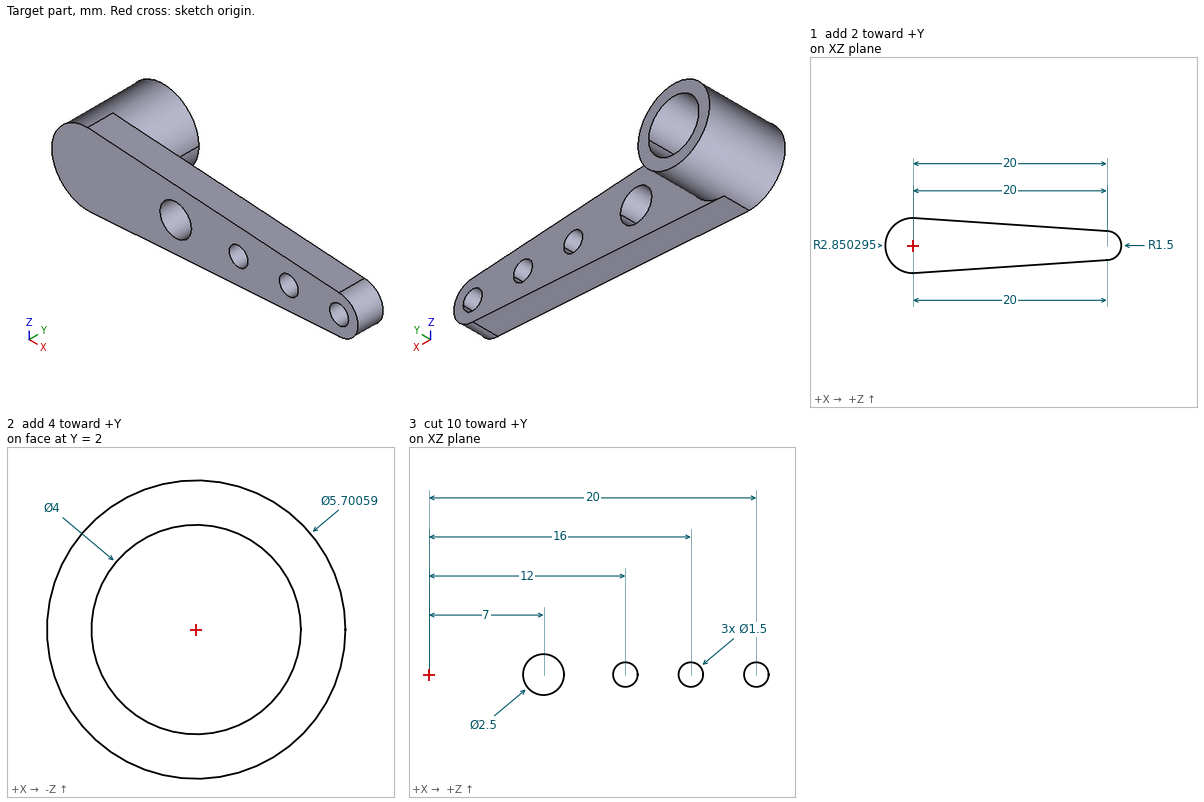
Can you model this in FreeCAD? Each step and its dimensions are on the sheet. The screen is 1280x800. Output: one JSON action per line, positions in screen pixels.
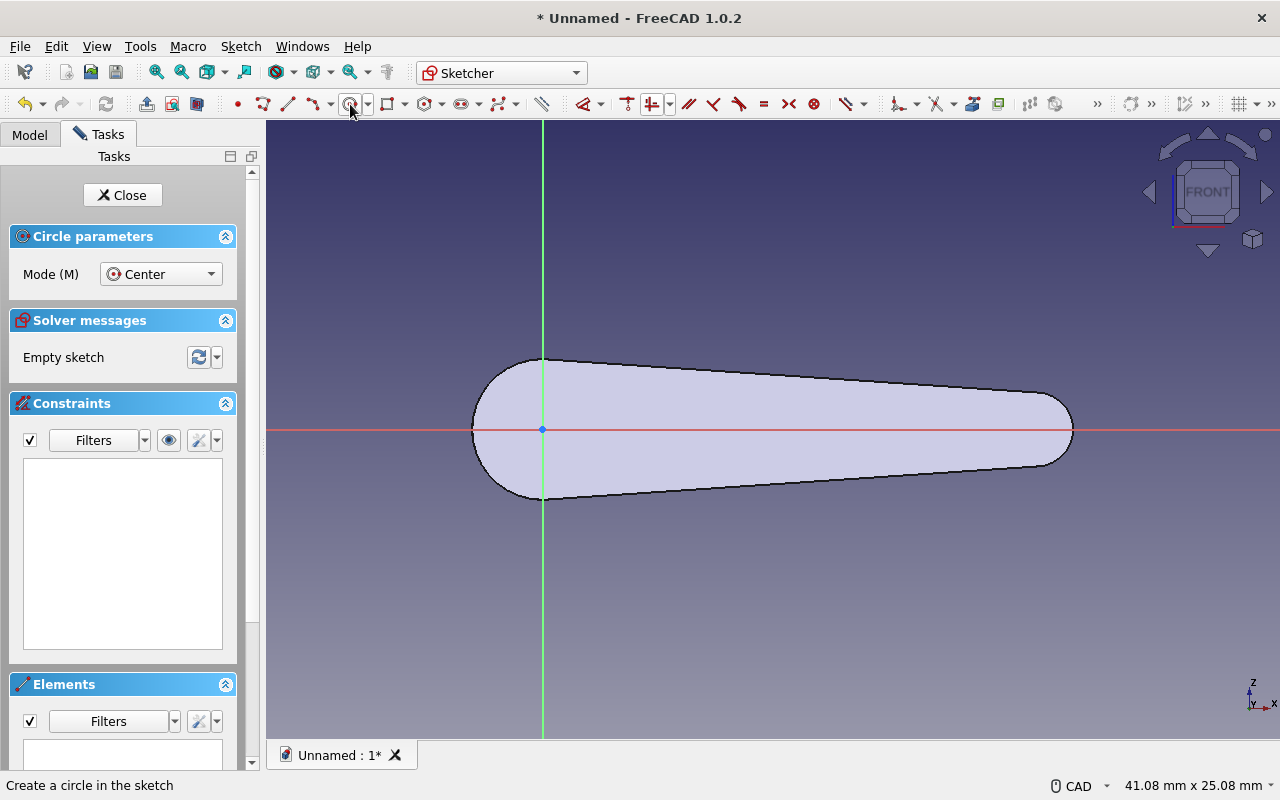
{"action": "scroll", "coordinate": [937, 430], "scroll_direction": "up", "scroll_amount": 2}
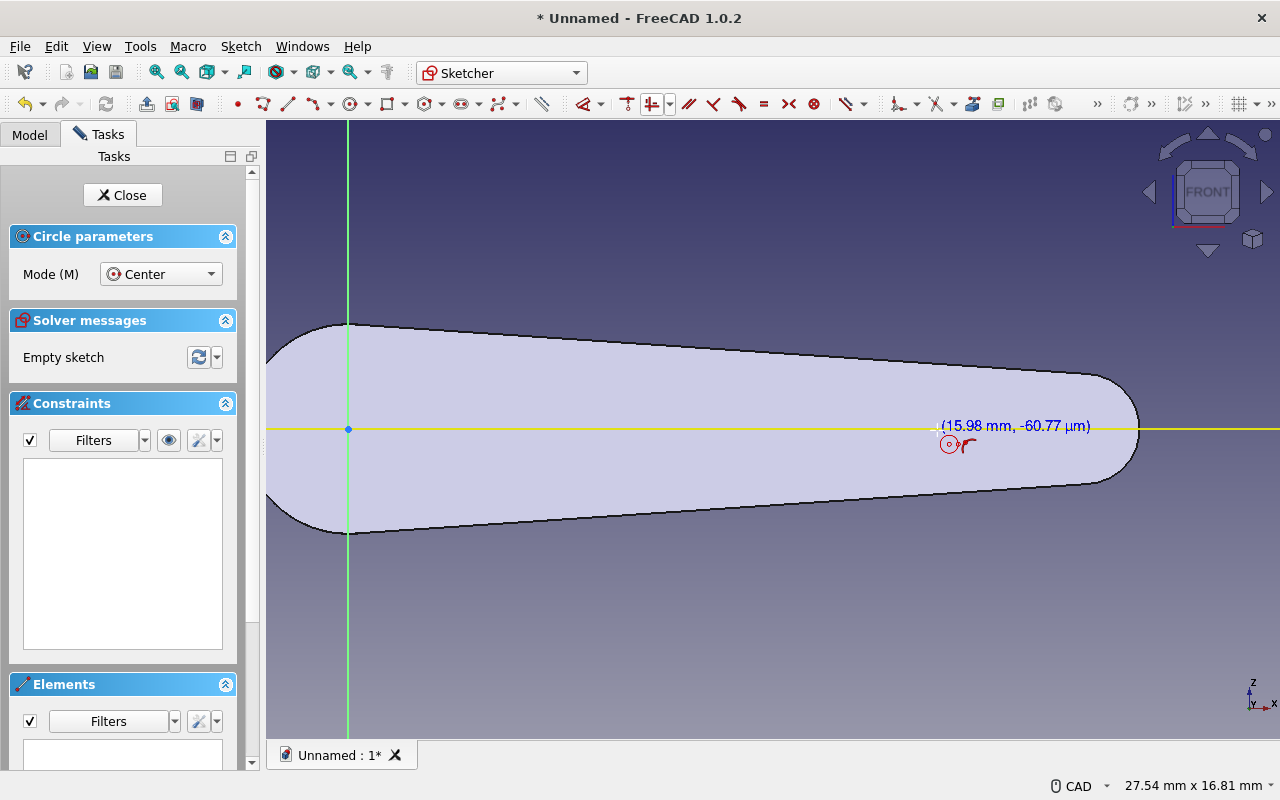
{"action": "left_click", "coordinate": [937, 429]}
{"action": "mouse_move", "coordinate": [957, 409]}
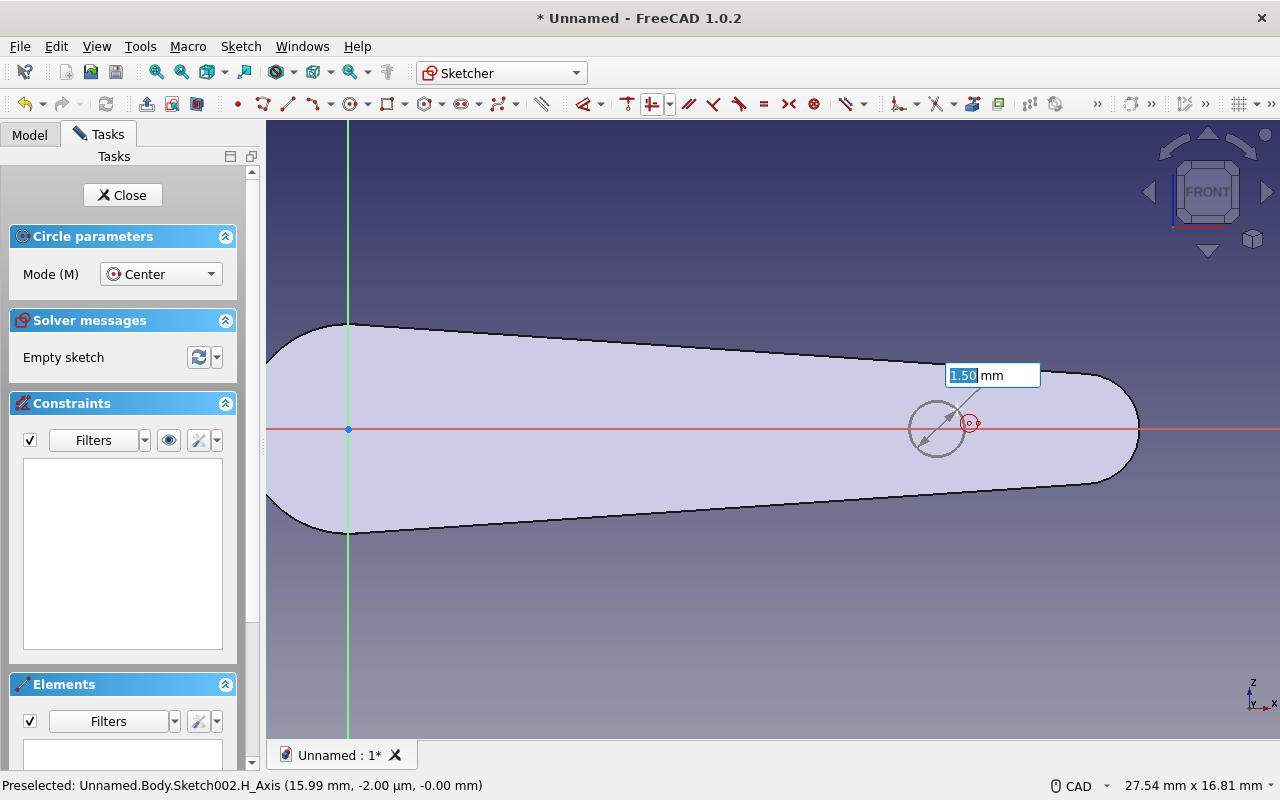
{"action": "type", "text": "1.5"}
{"action": "key", "text": "Return"}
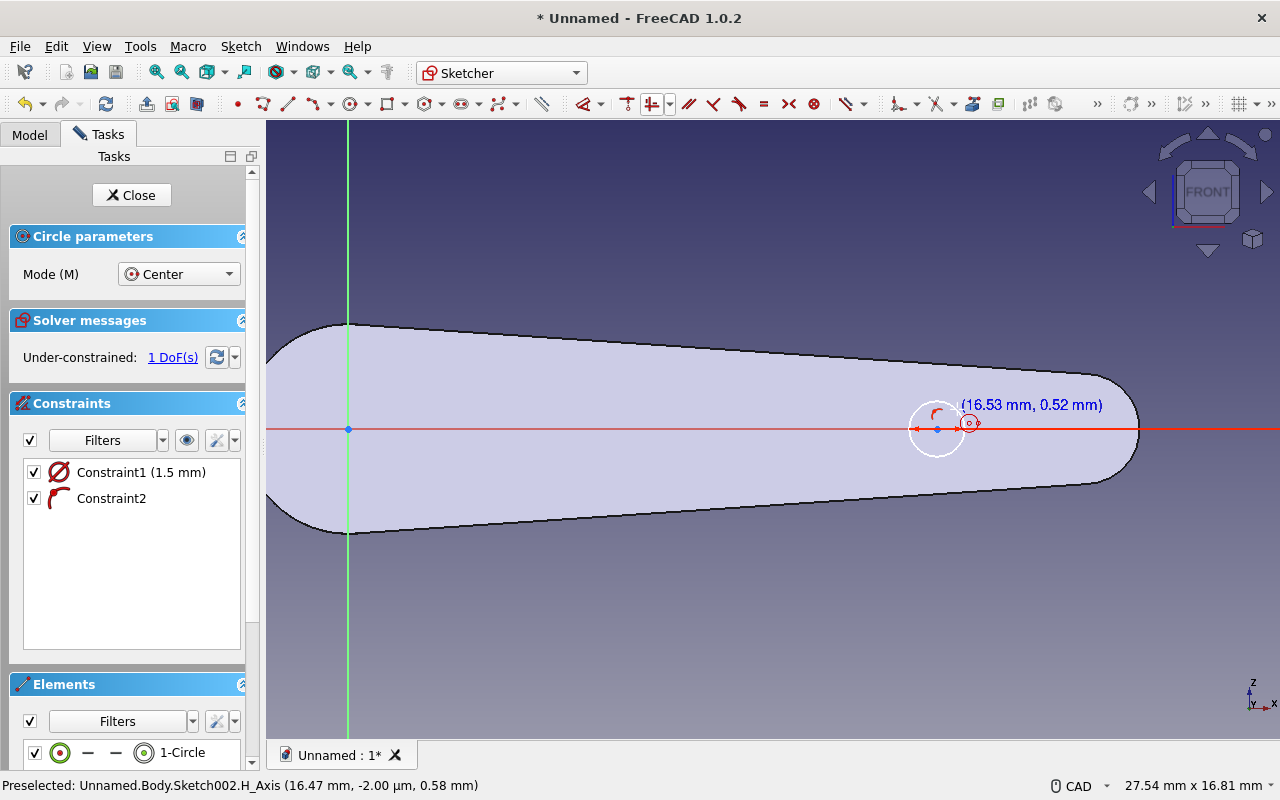
{"action": "left_click", "coordinate": [790, 429]}
{"action": "mouse_move", "coordinate": [810, 409]}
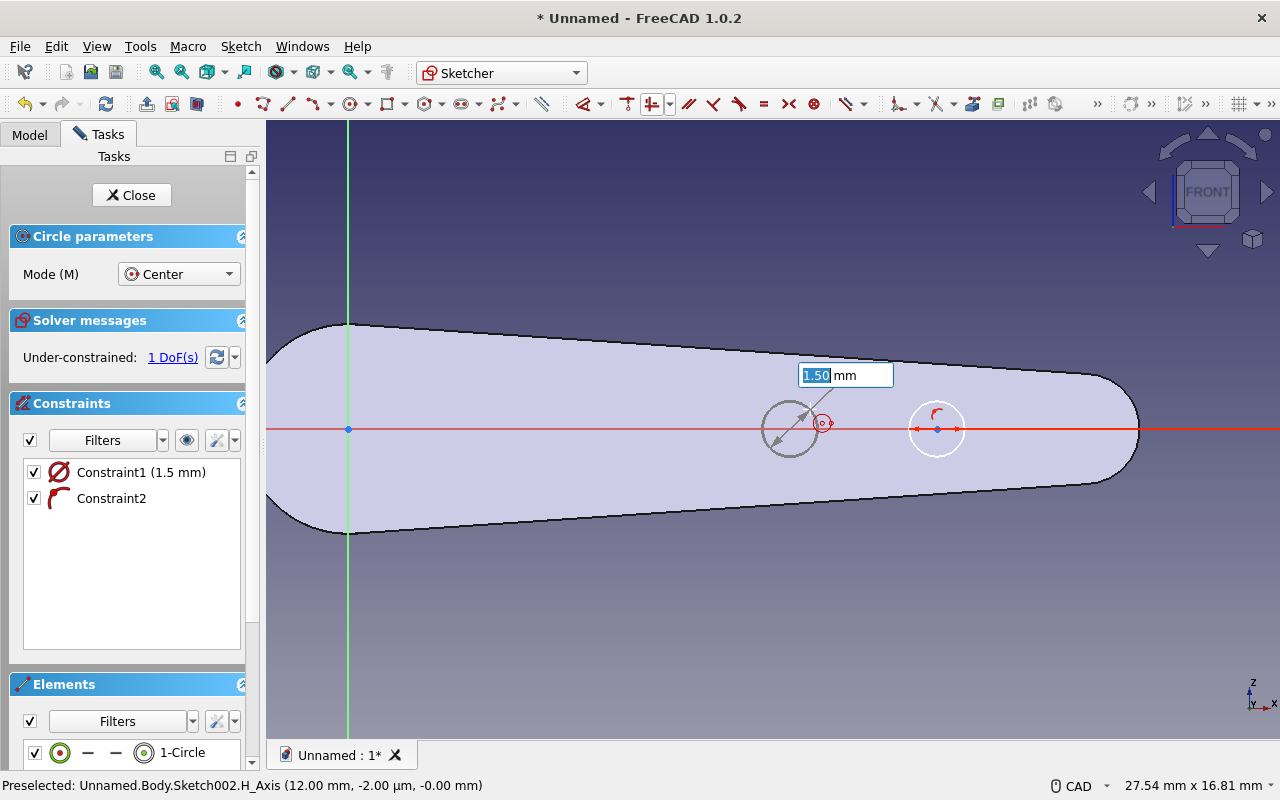
{"action": "type", "text": "1.5"}
{"action": "key", "text": "Return"}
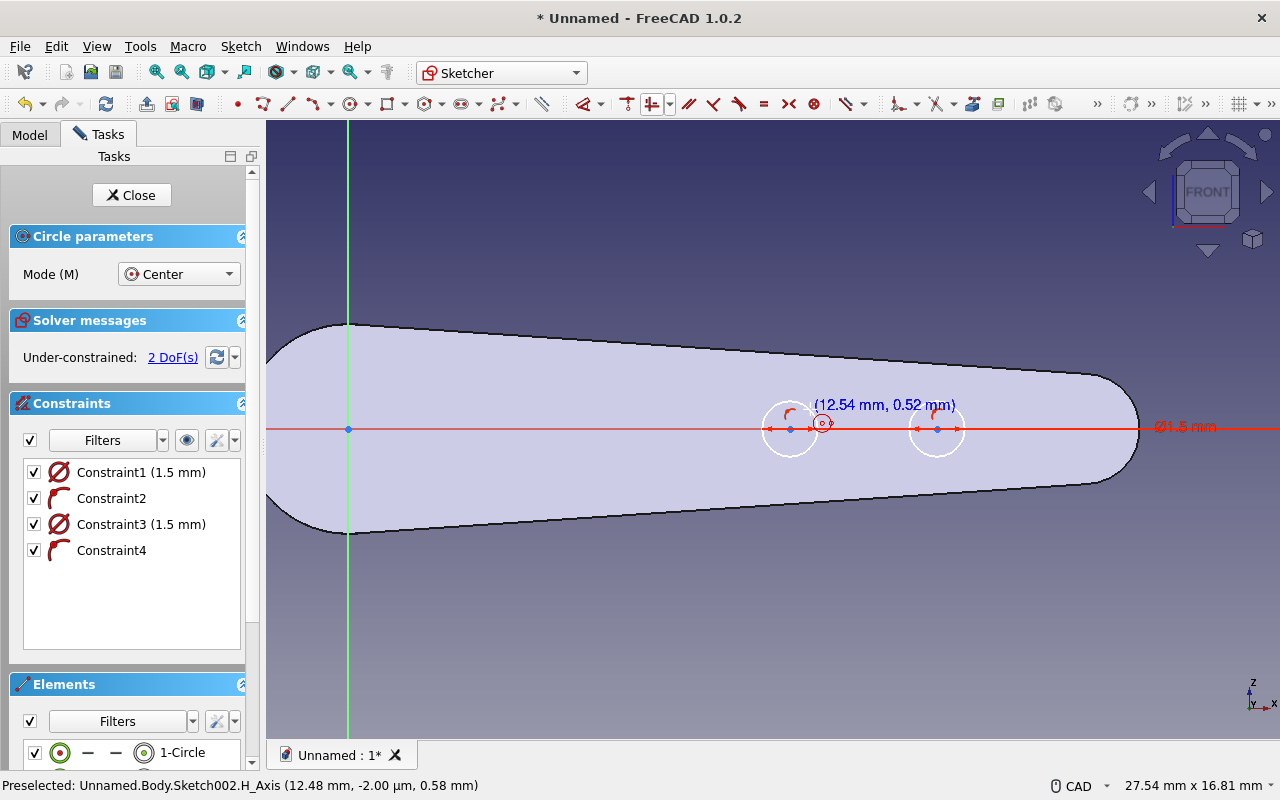
{"action": "left_click", "coordinate": [606, 429]}
{"action": "mouse_move", "coordinate": [638, 396]}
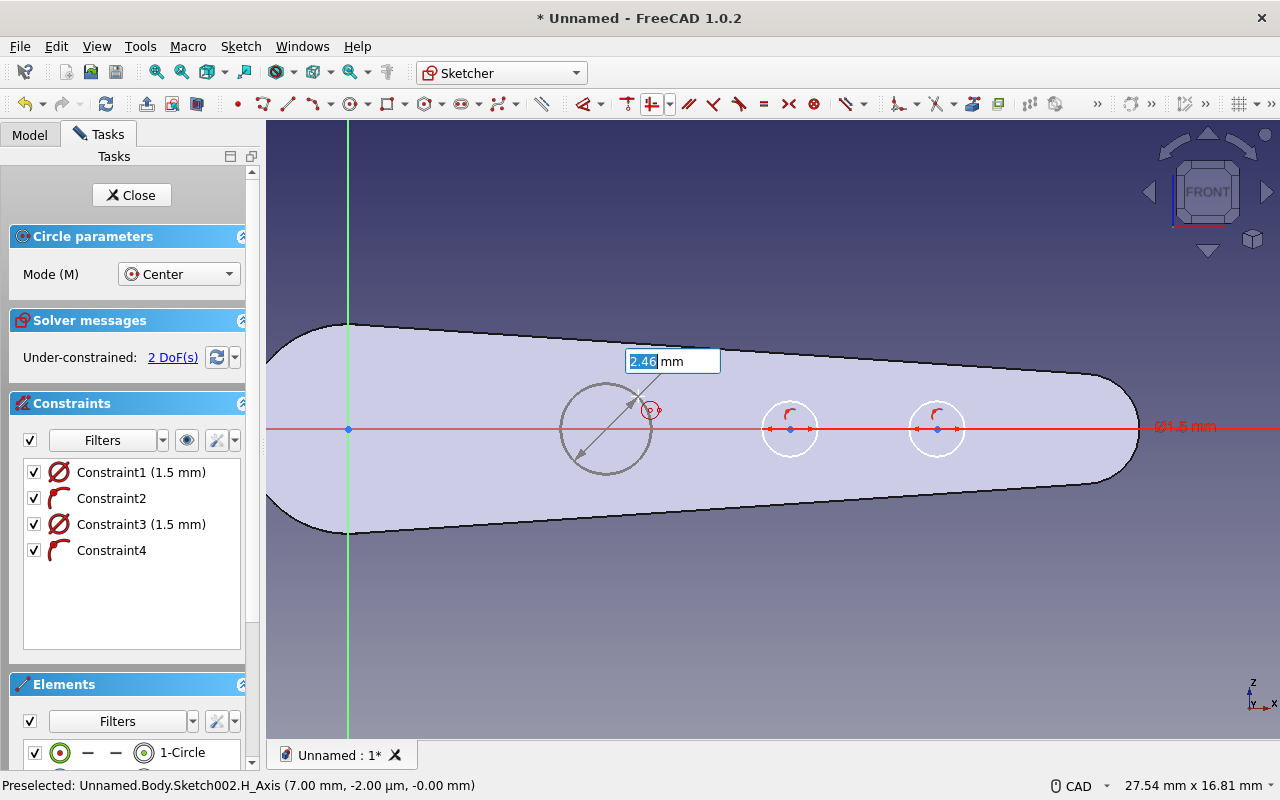
{"action": "type", "text": "2.5"}
{"action": "key", "text": "Return"}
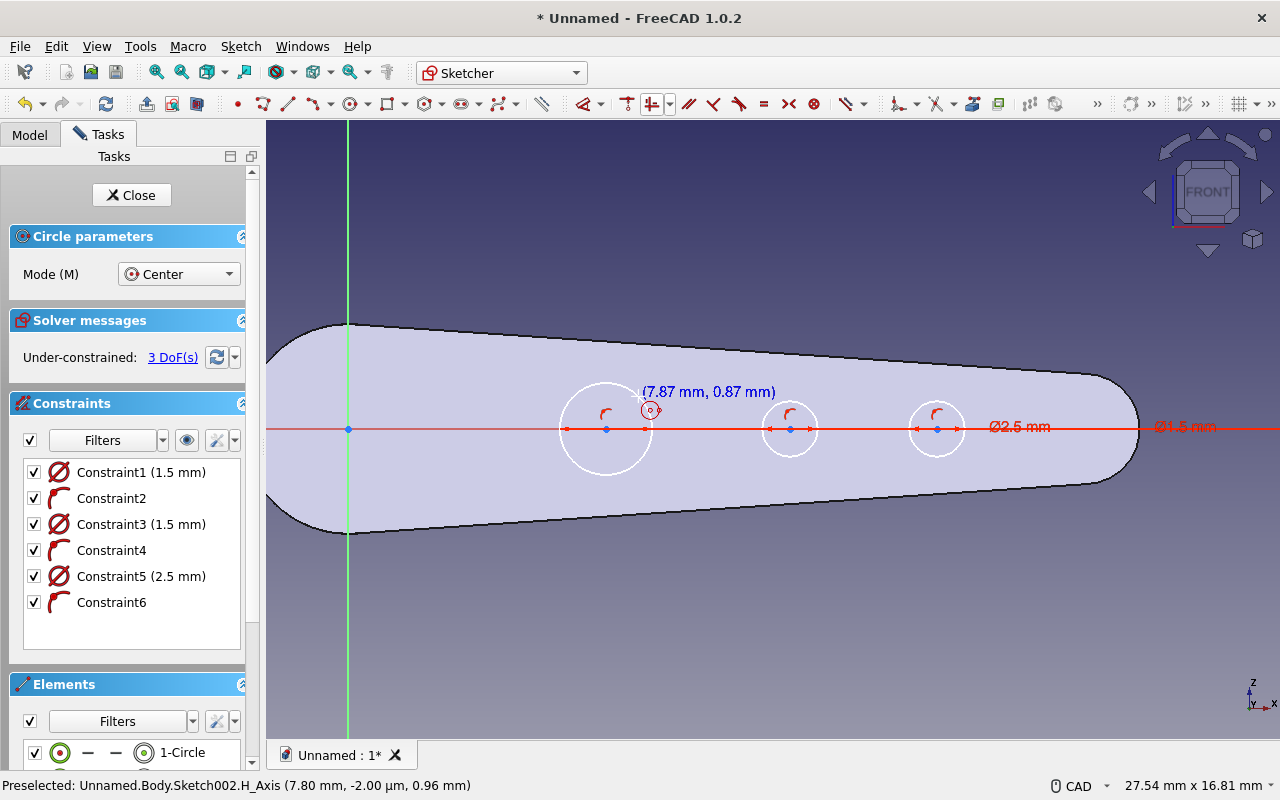
{"action": "left_click", "coordinate": [1085, 429]}
{"action": "mouse_move", "coordinate": [1104, 409]}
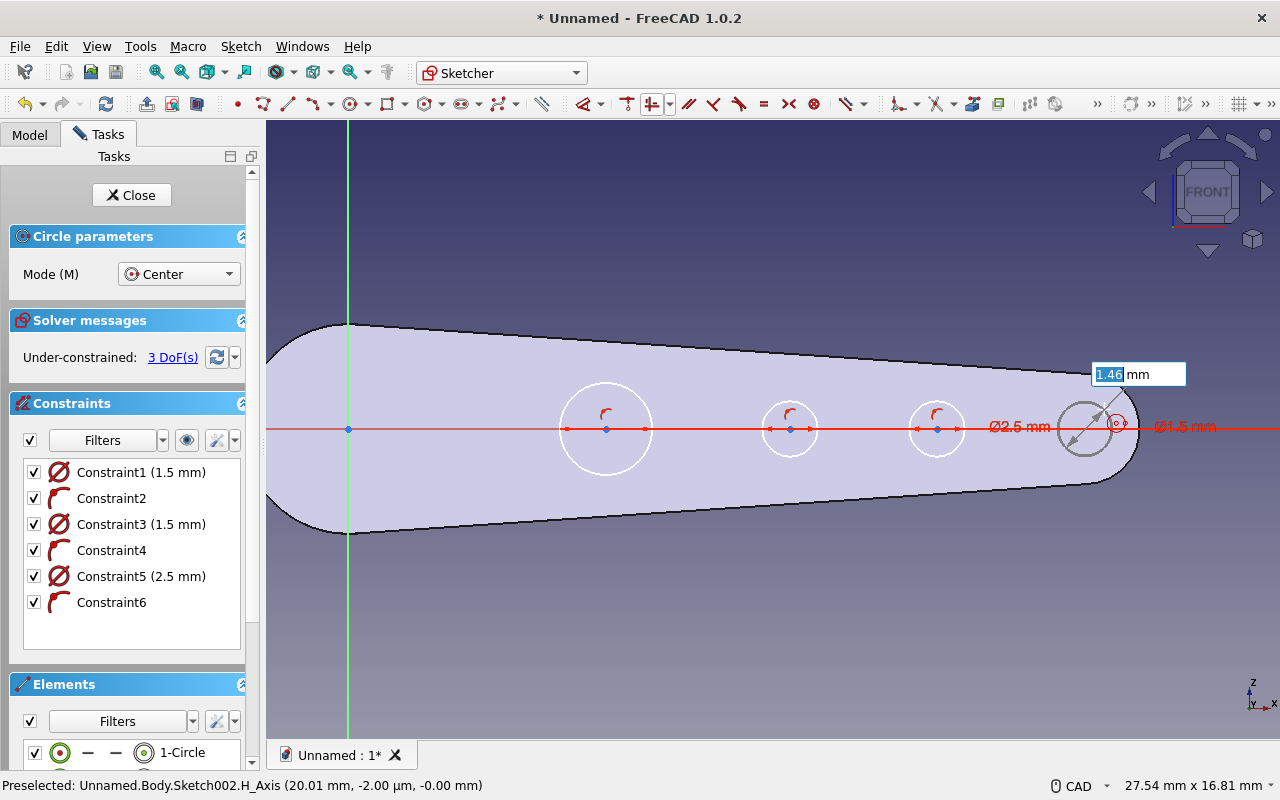
{"action": "type", "text": "1.5"}
{"action": "key", "text": "Return"}
{"action": "key", "text": "Escape"}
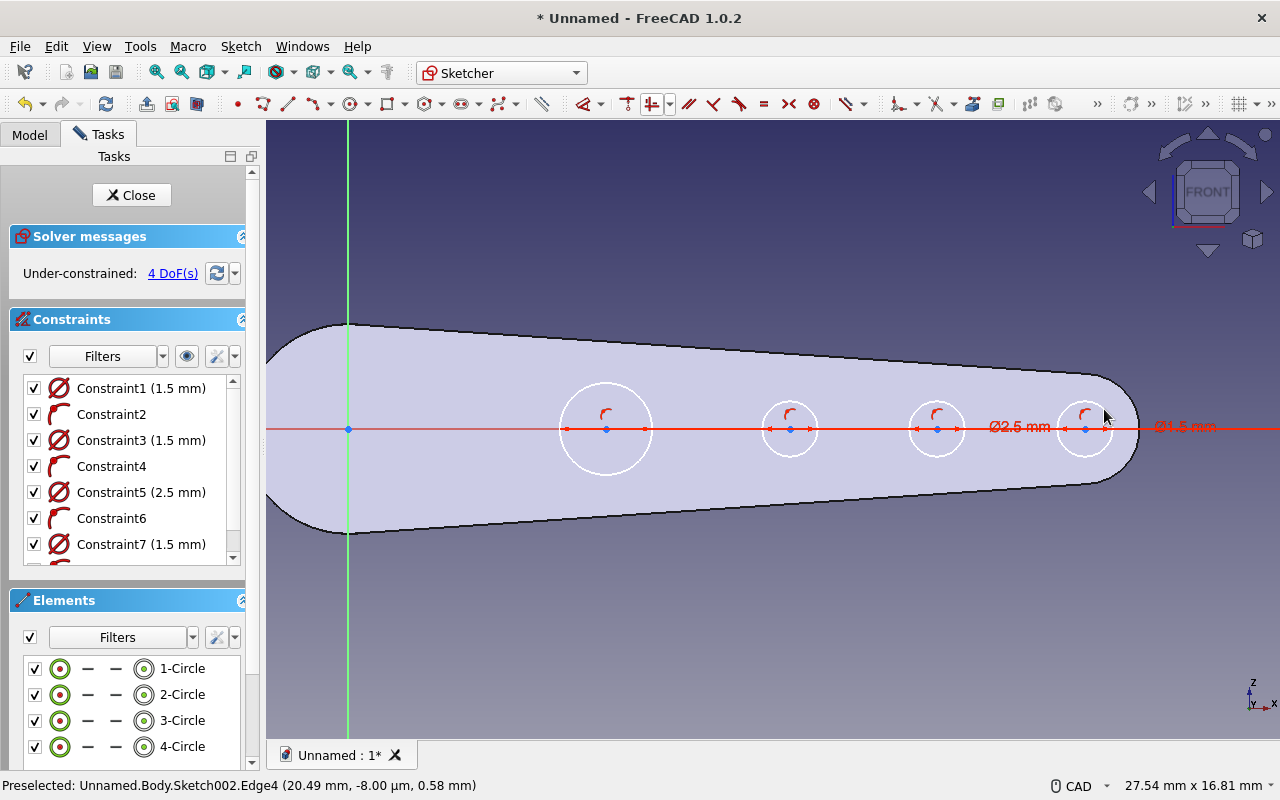
{"action": "left_click", "coordinate": [582, 104]}